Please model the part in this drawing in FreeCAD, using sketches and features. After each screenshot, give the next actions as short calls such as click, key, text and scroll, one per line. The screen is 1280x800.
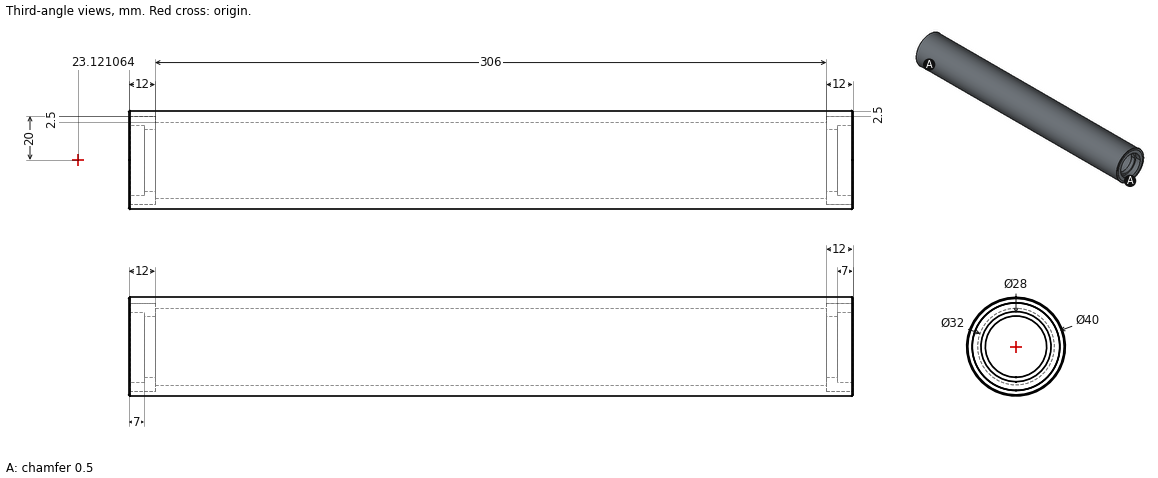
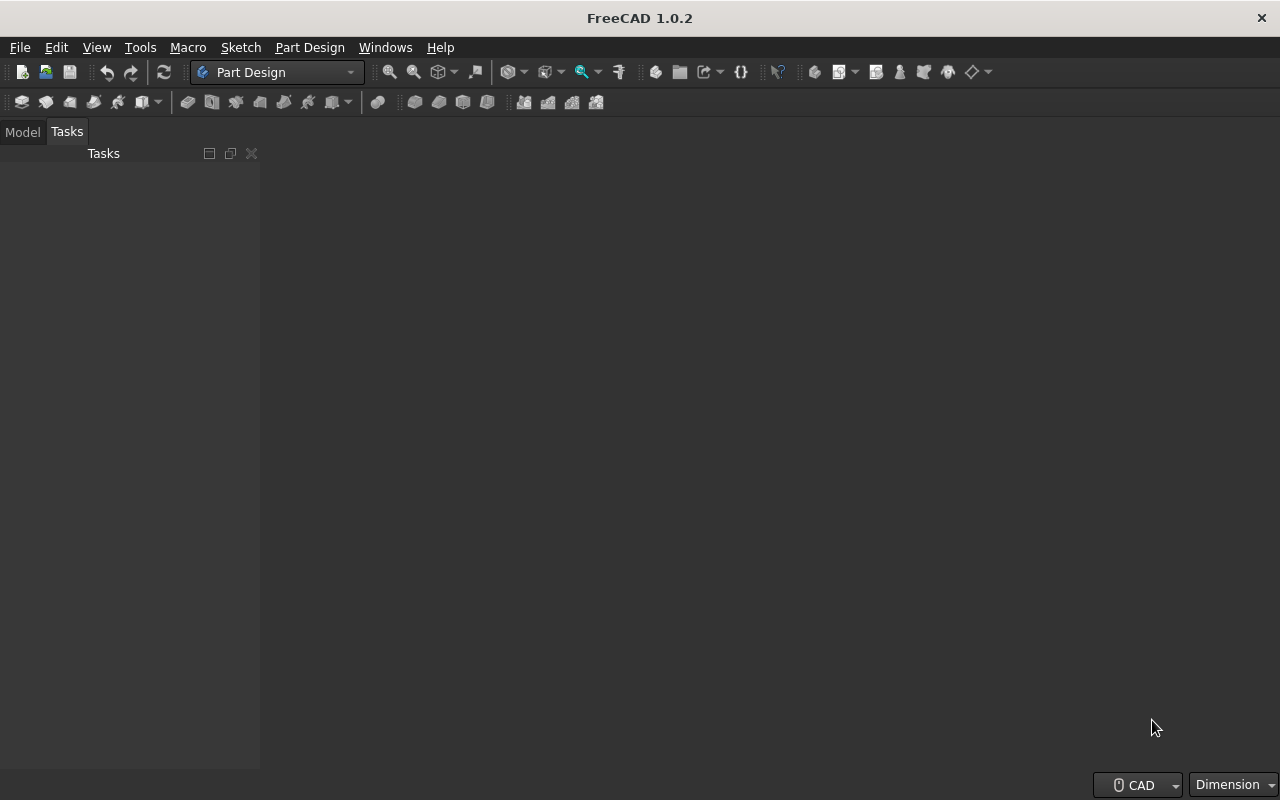
click(22, 72)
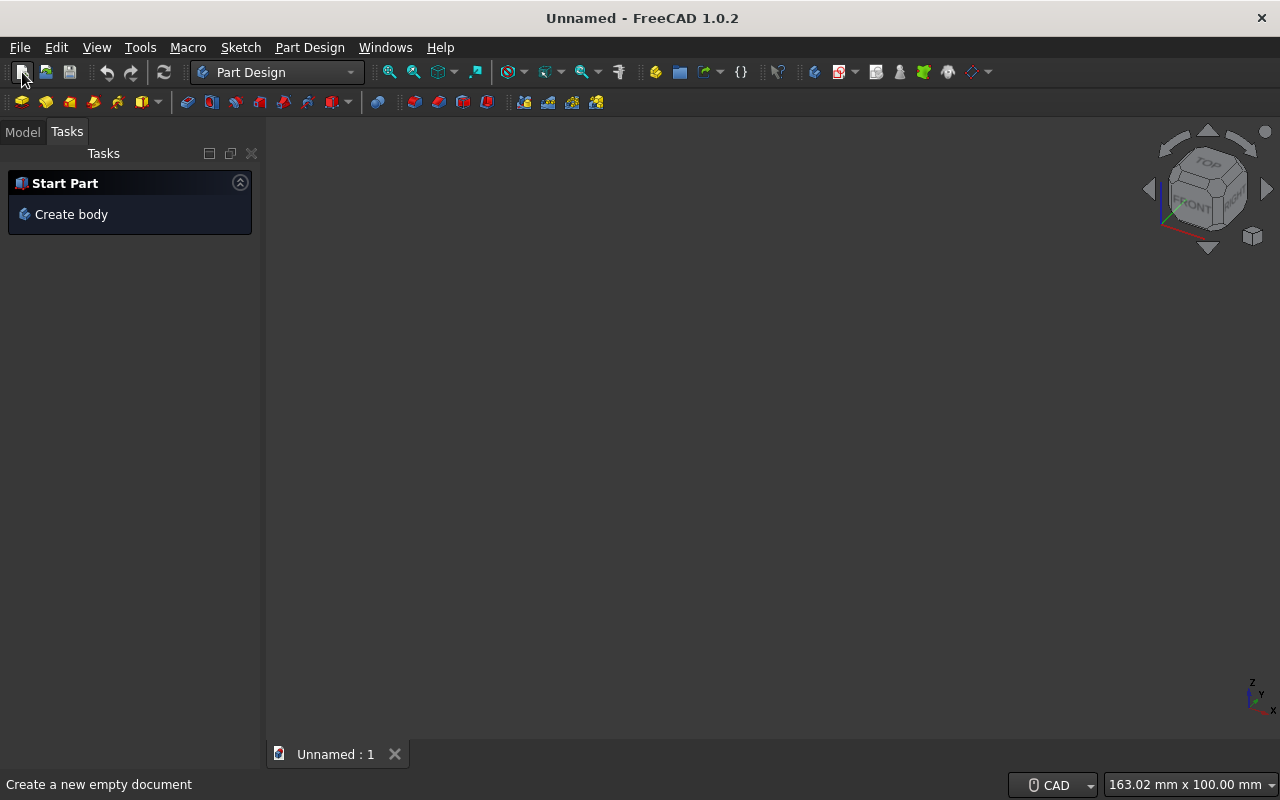
click(840, 72)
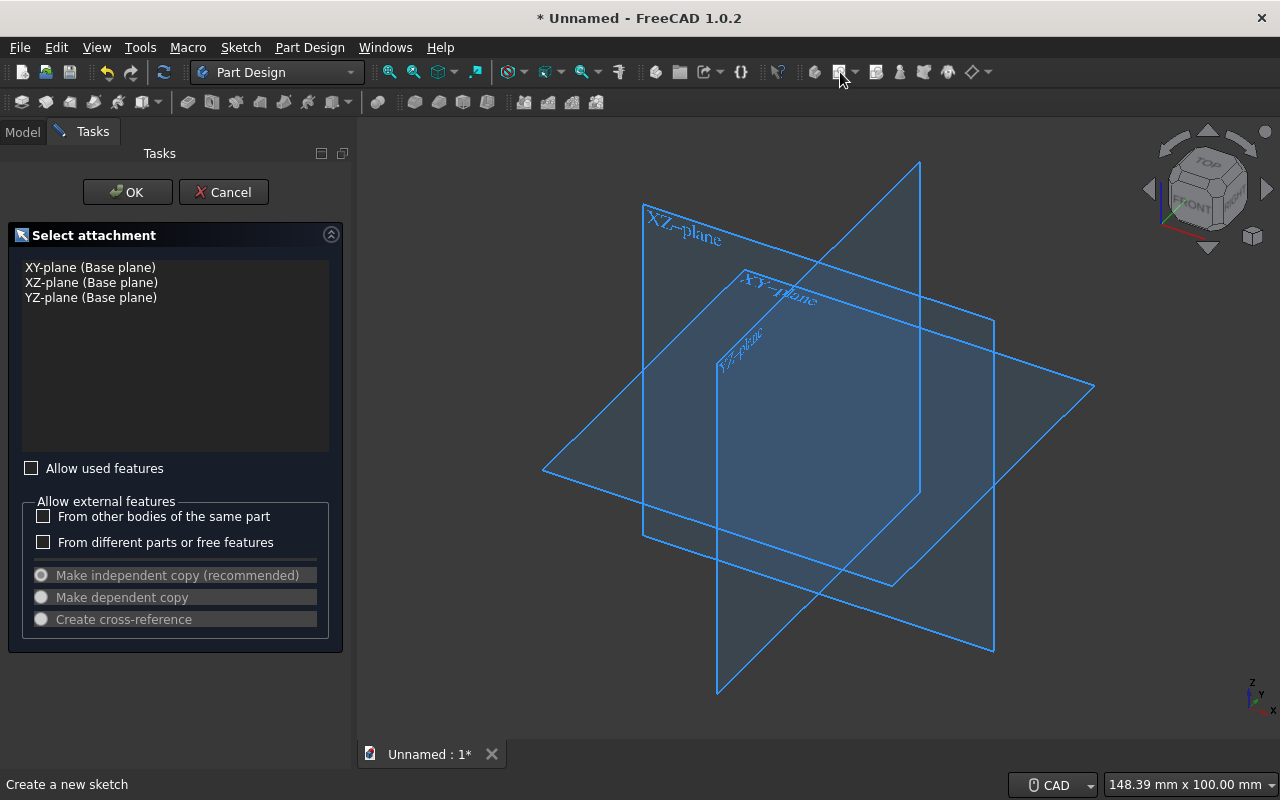
click(82, 268)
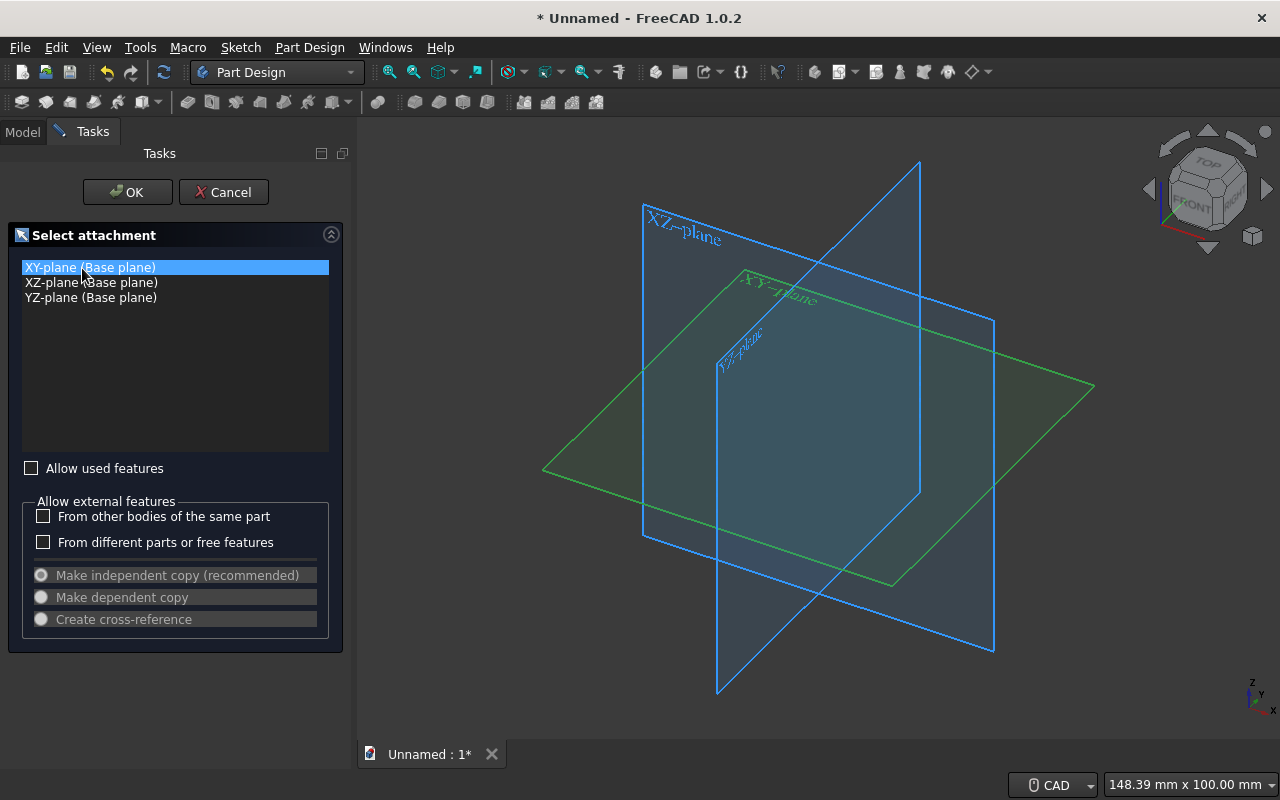
click(128, 192)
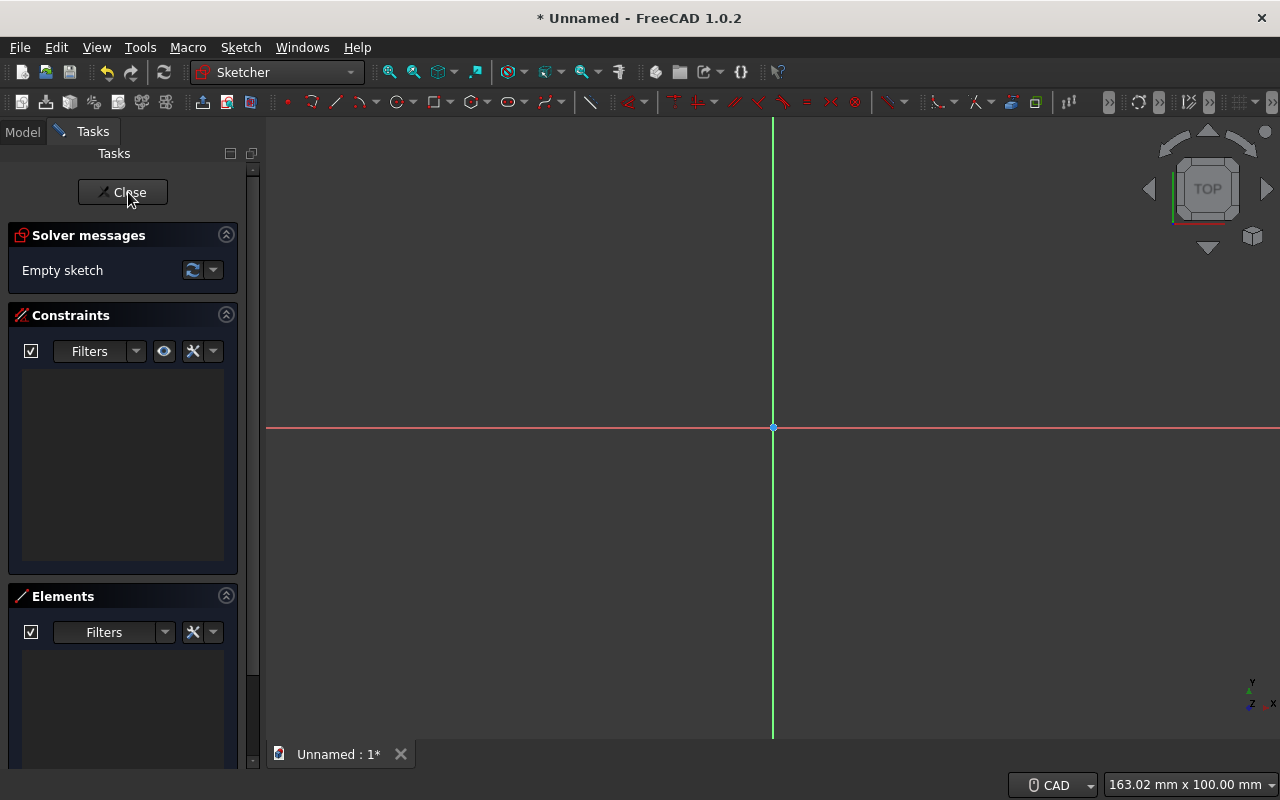
scroll(323, 451, down, 7)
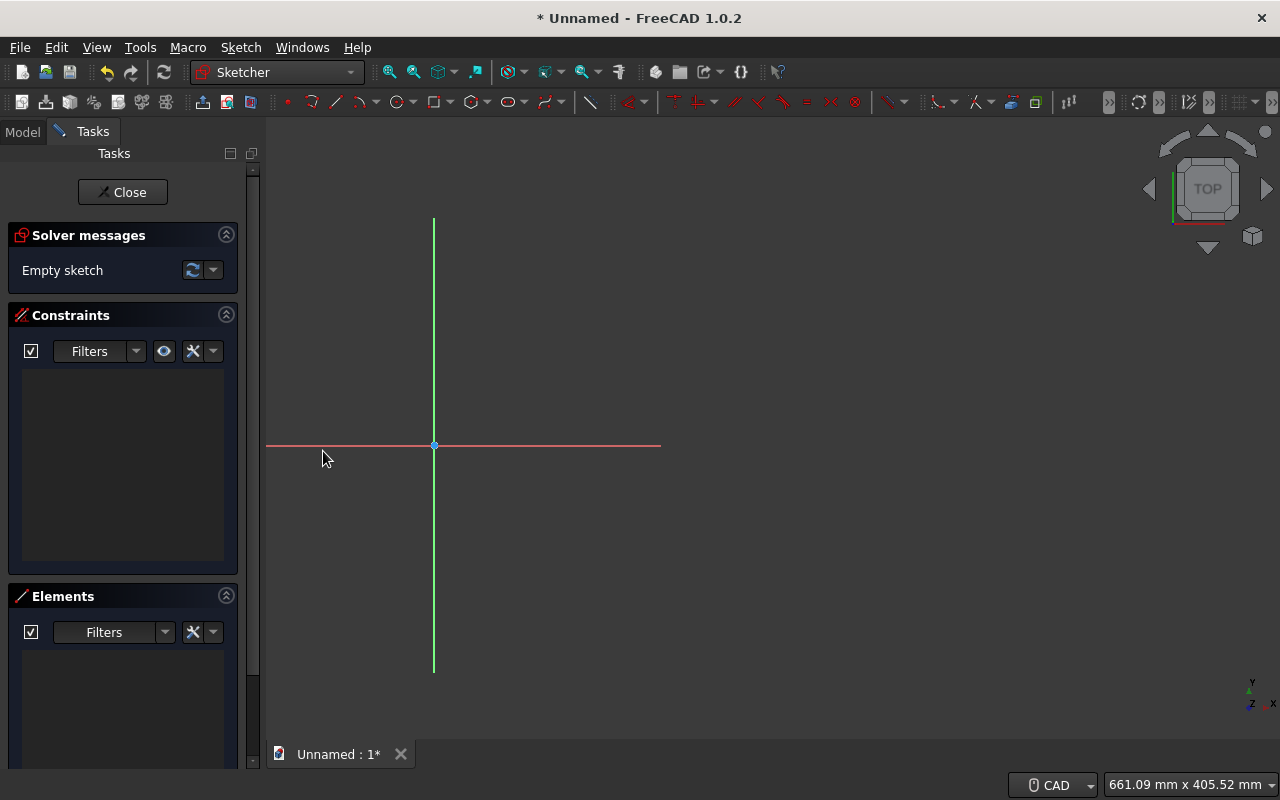
click(312, 102)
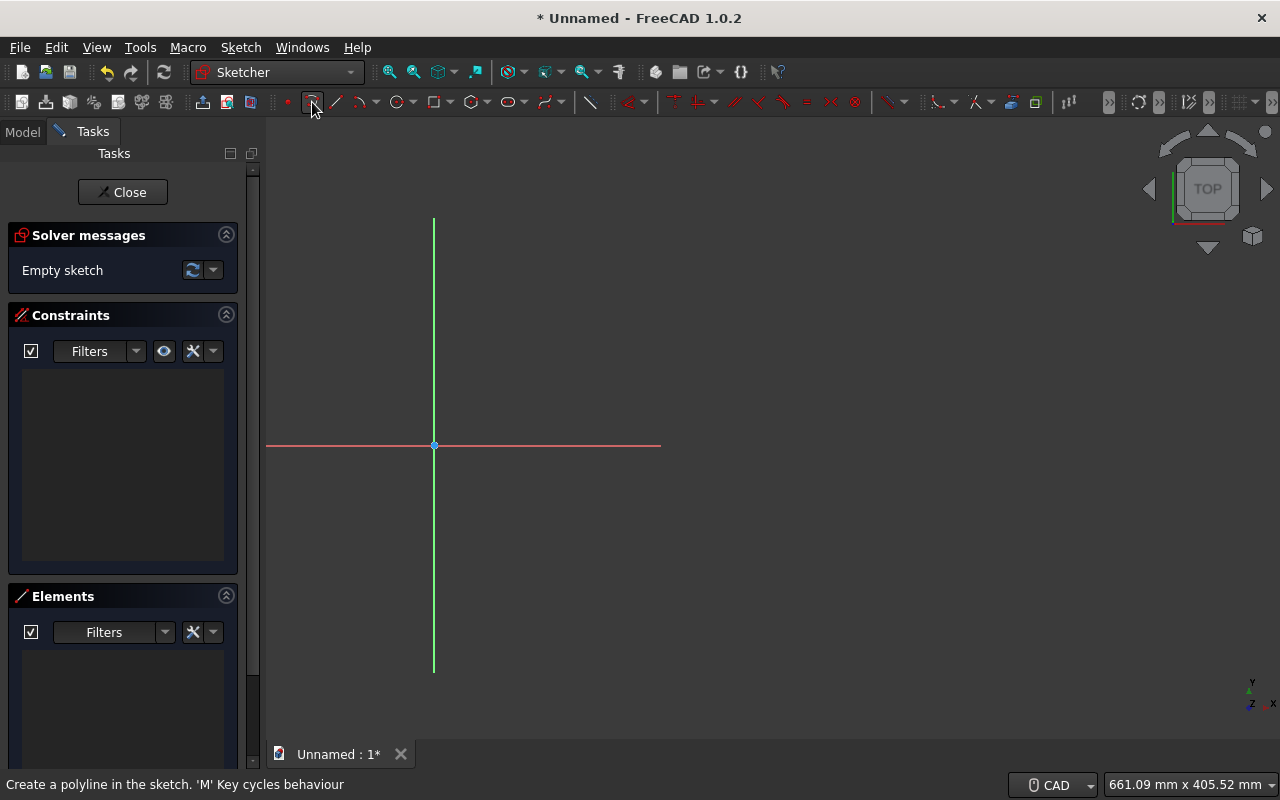
click(469, 415)
click(488, 415)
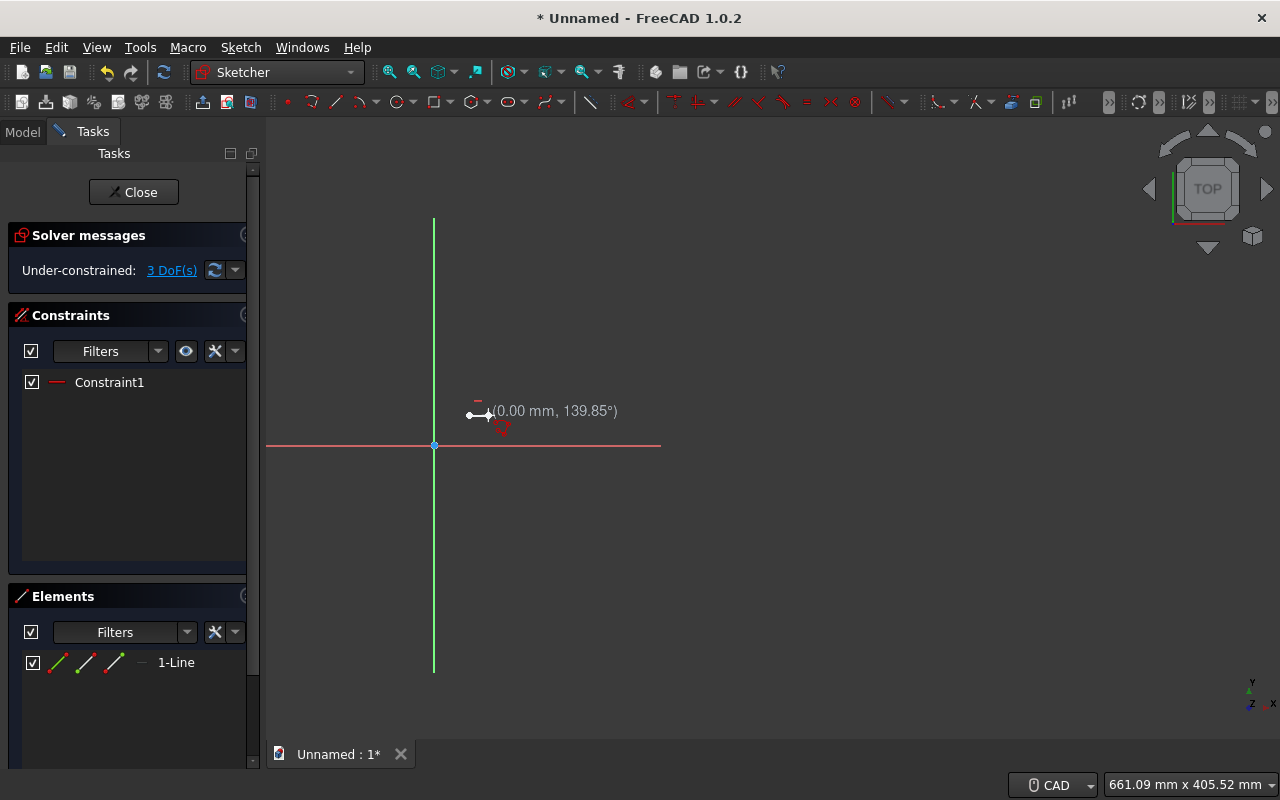
scroll(488, 419, up, 8)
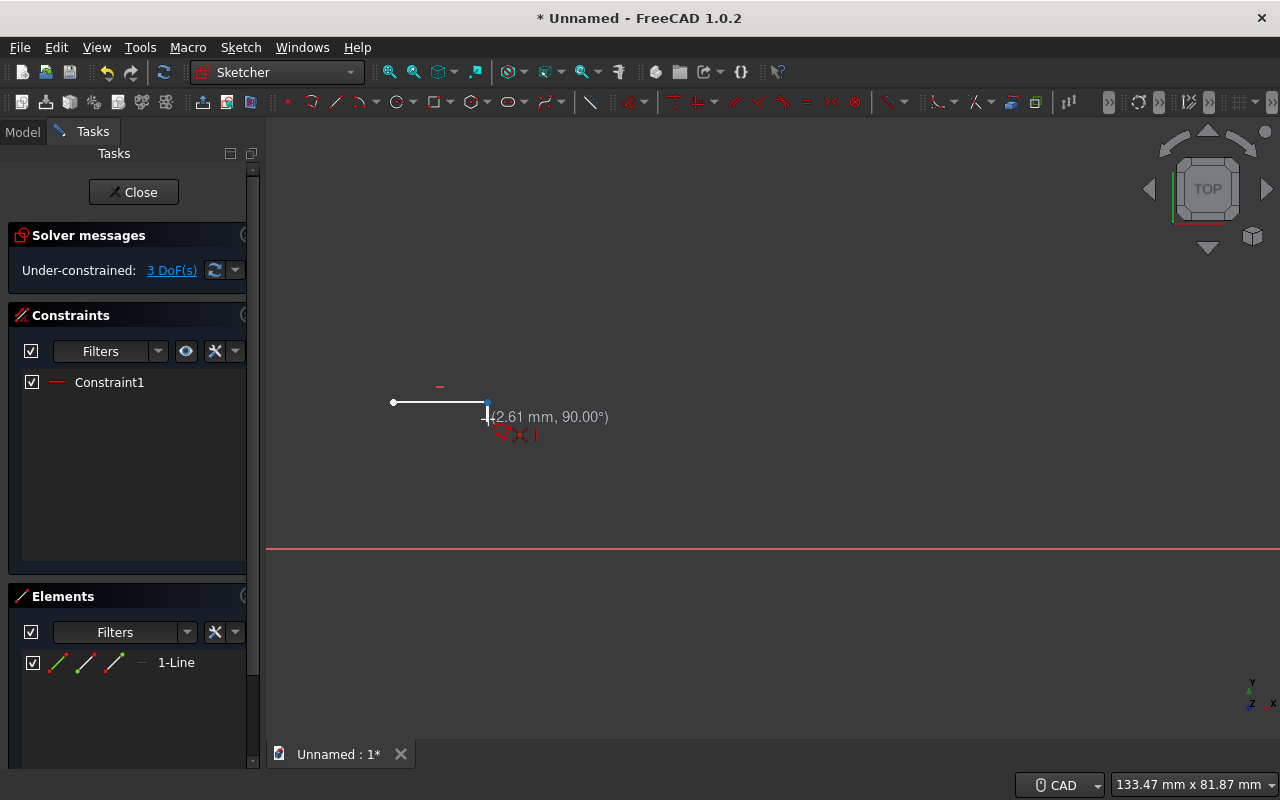
click(487, 417)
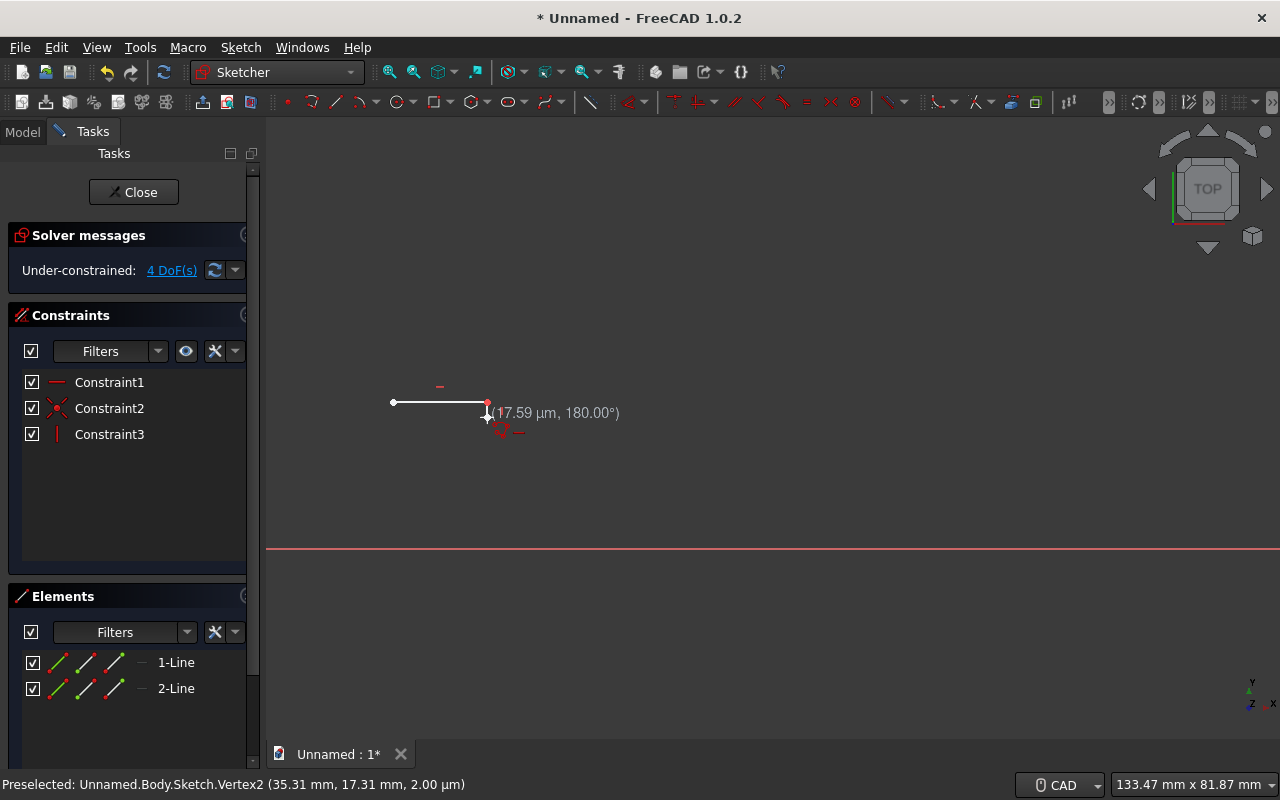
scroll(488, 419, down, 8)